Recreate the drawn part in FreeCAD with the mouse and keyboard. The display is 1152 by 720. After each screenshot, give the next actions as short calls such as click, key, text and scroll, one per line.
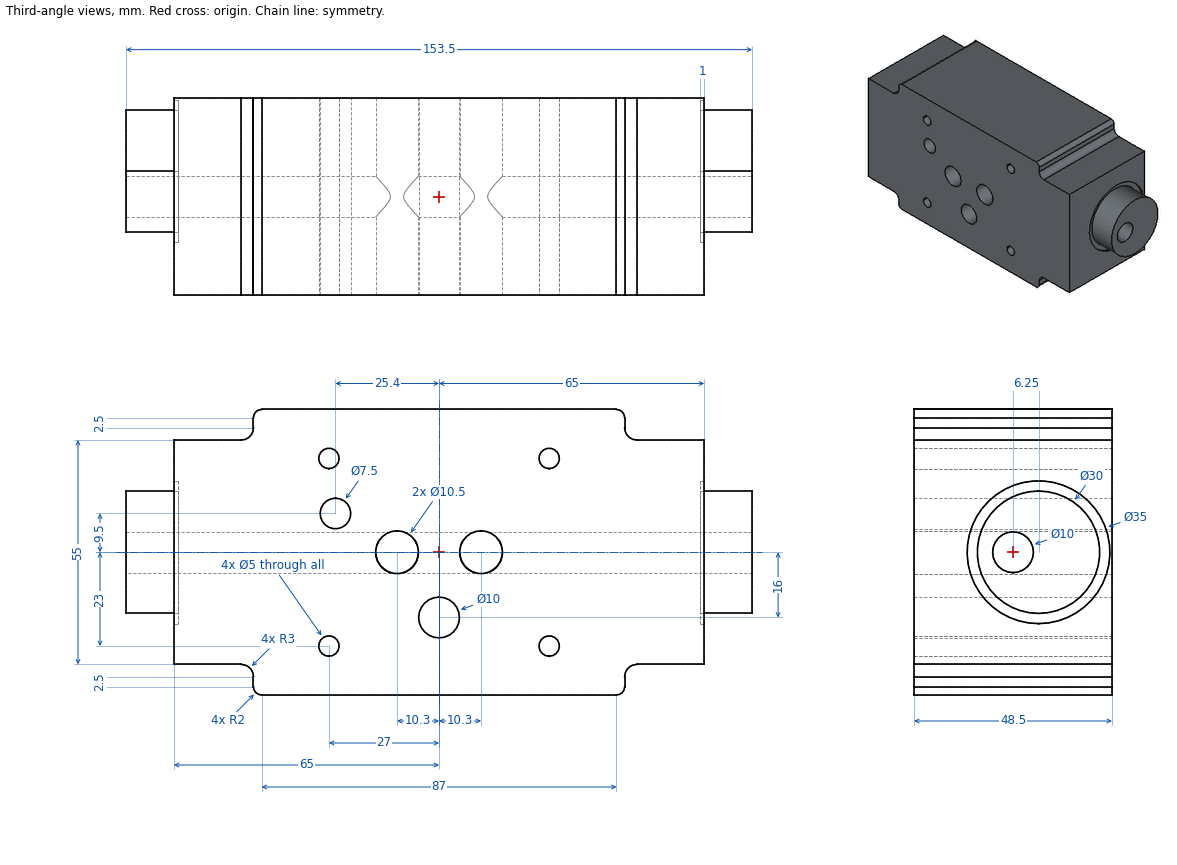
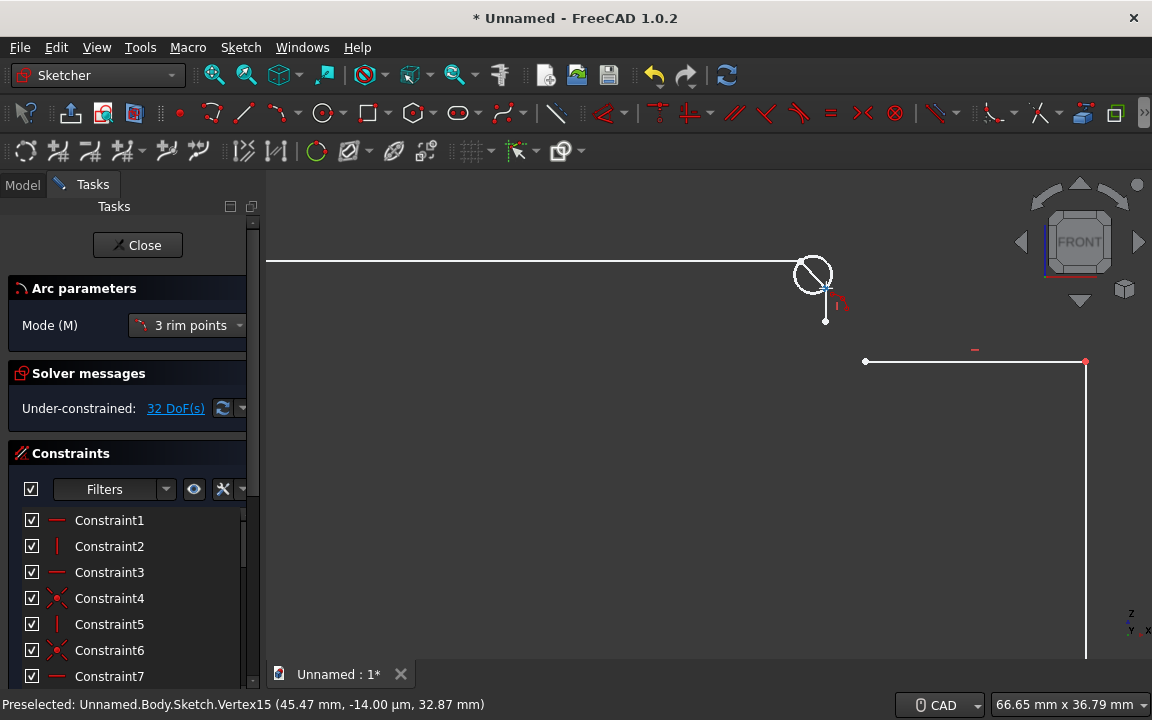
scroll(818, 268, up, 4)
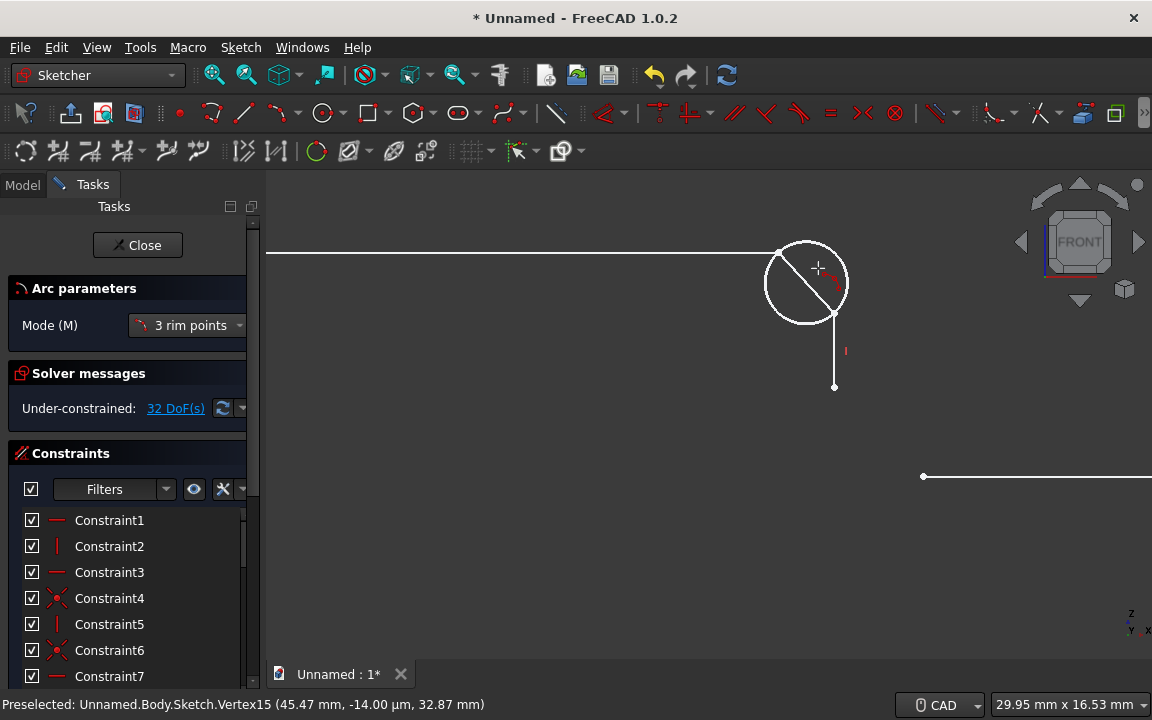
click(818, 268)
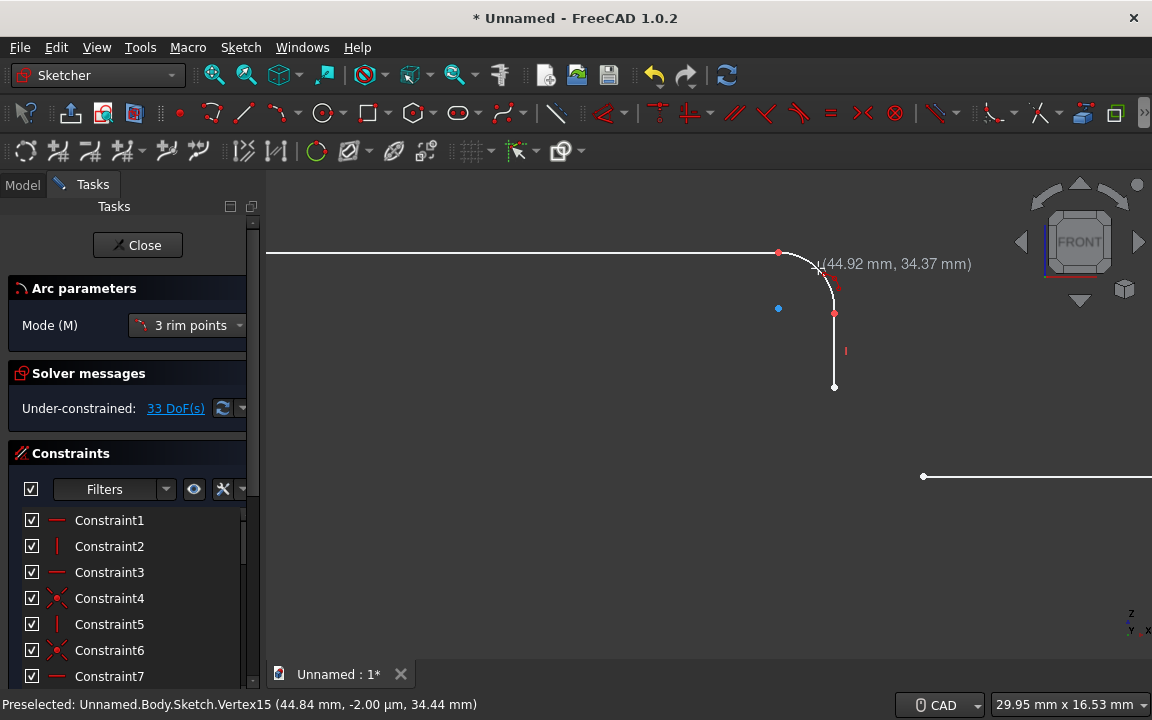
click(834, 387)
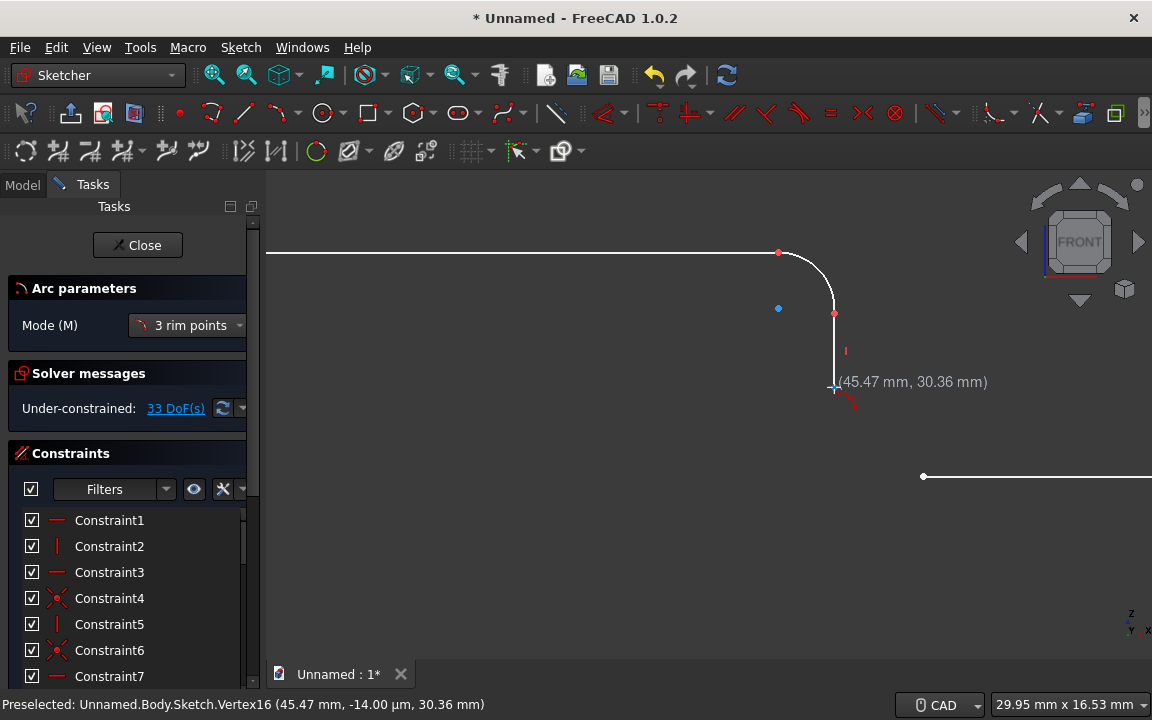
scroll(821, 278, down, 10)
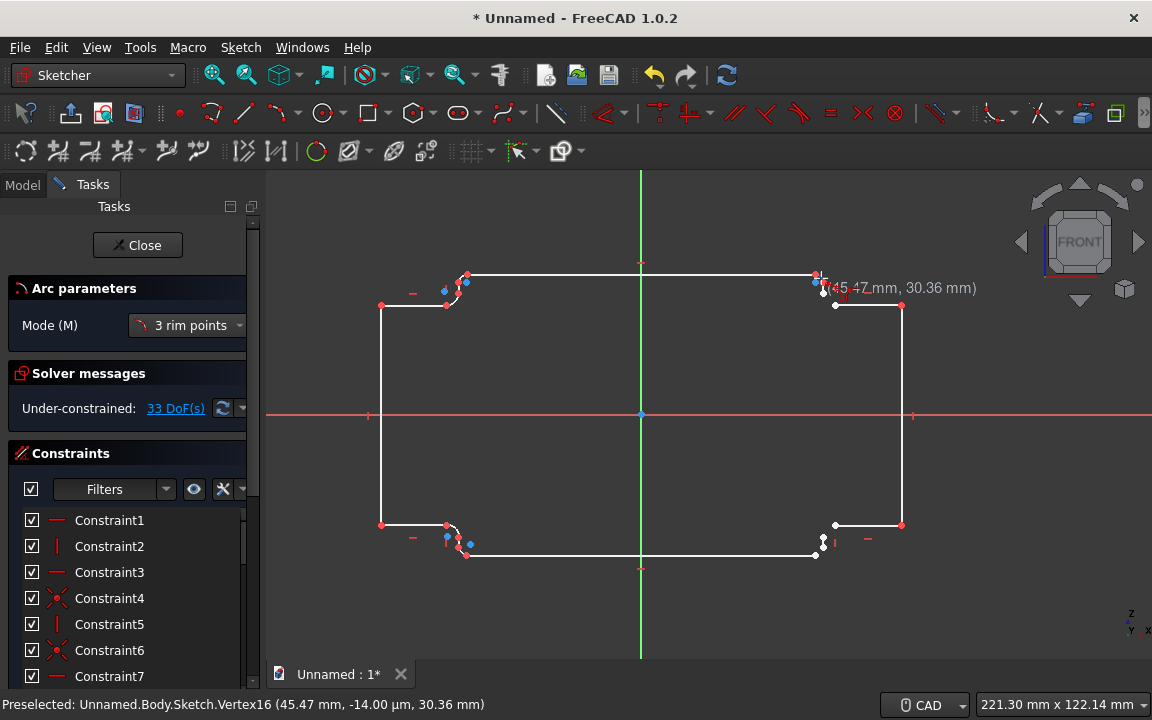
click(835, 305)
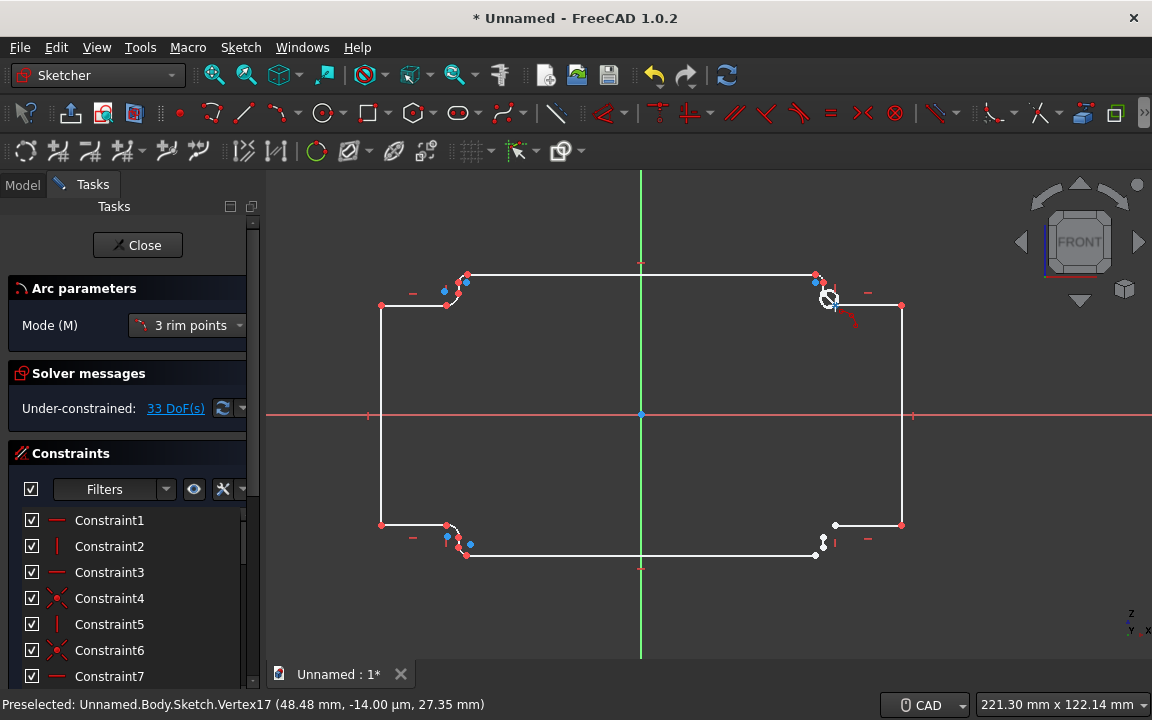
scroll(827, 301, up, 8)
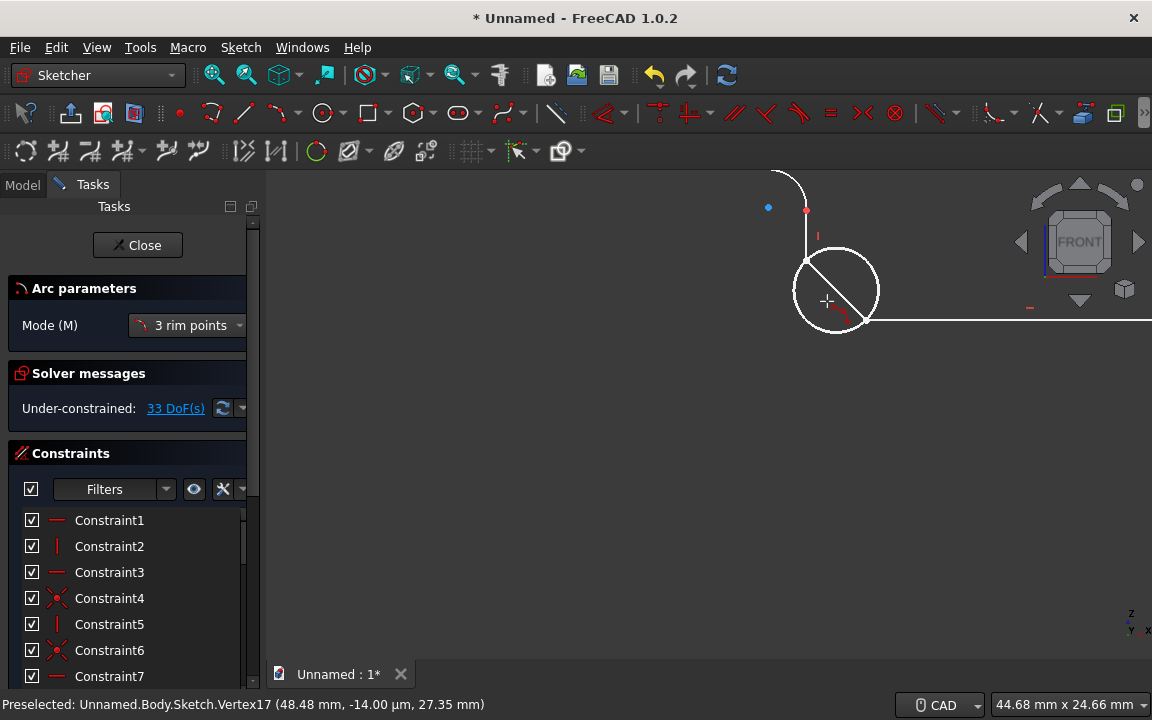
click(824, 300)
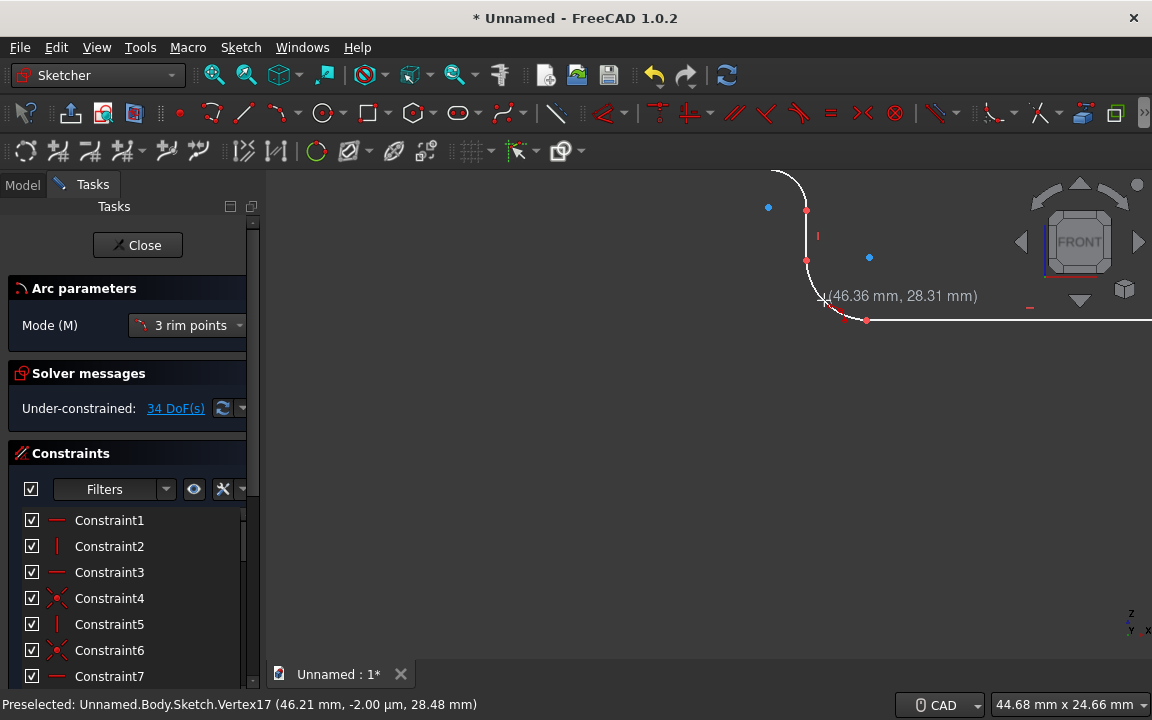
scroll(827, 301, down, 8)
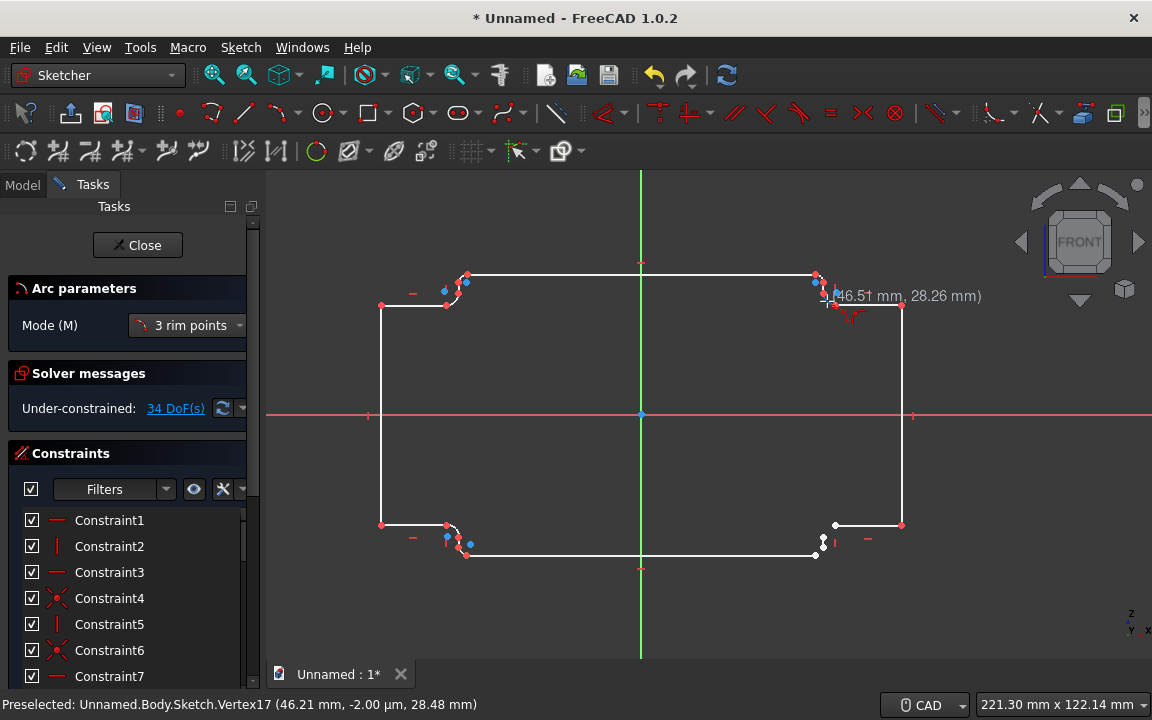
click(835, 526)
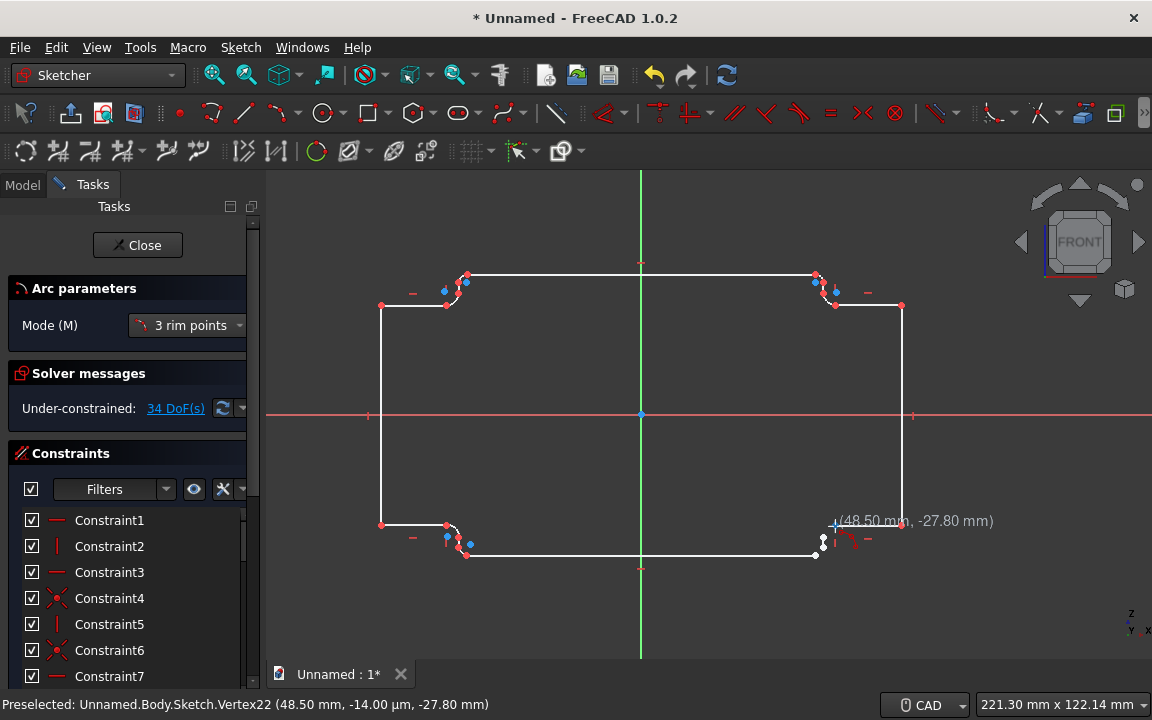
scroll(823, 537, up, 6)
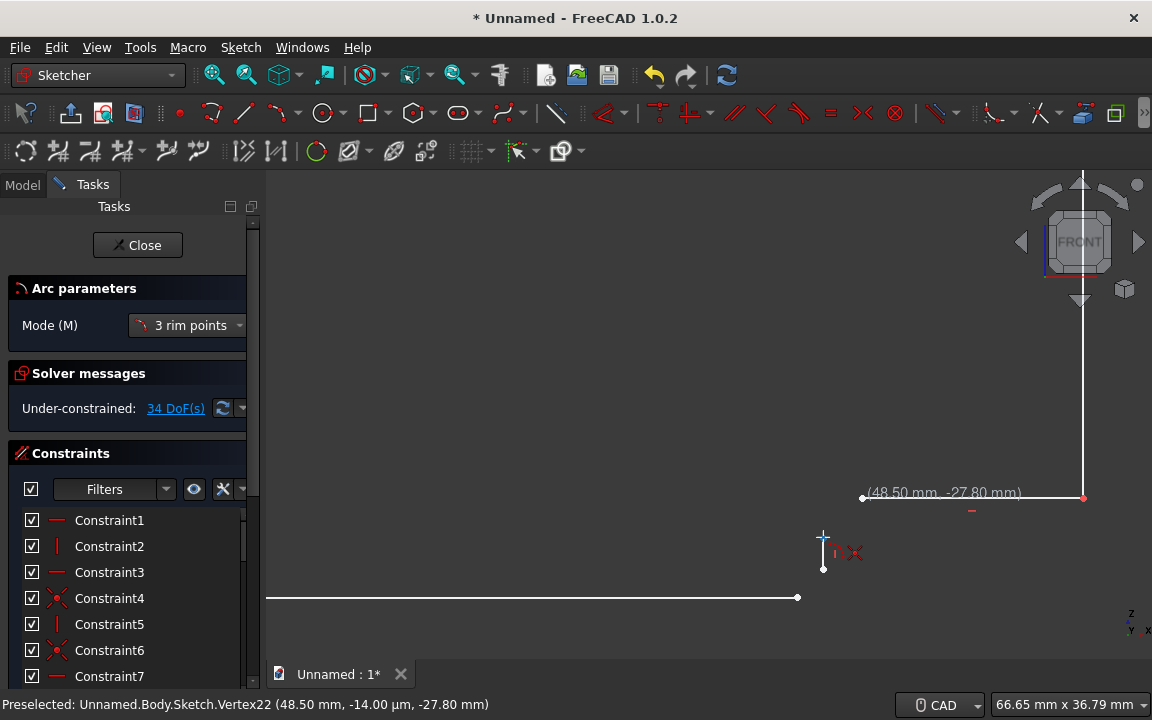
click(823, 538)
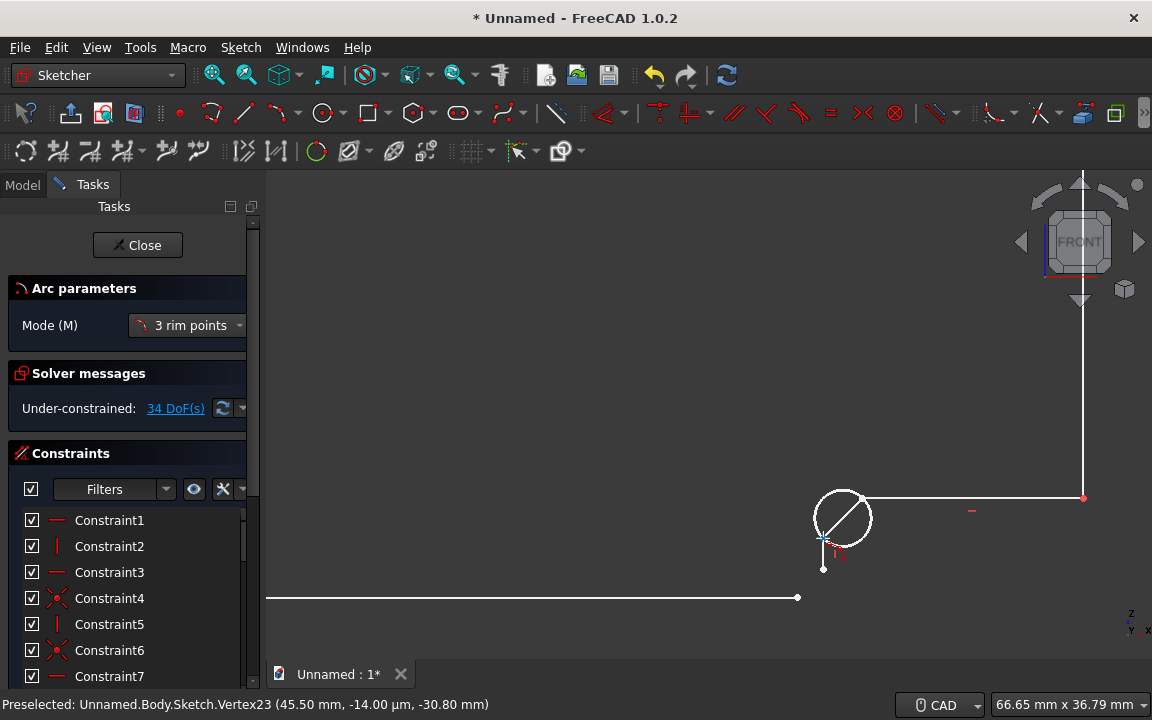
scroll(835, 506, up, 2)